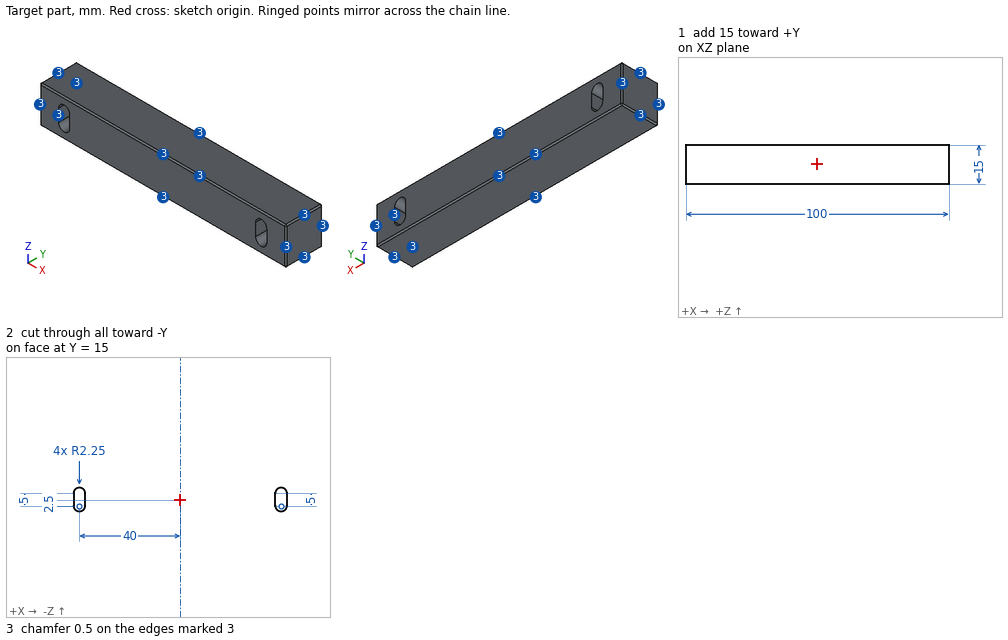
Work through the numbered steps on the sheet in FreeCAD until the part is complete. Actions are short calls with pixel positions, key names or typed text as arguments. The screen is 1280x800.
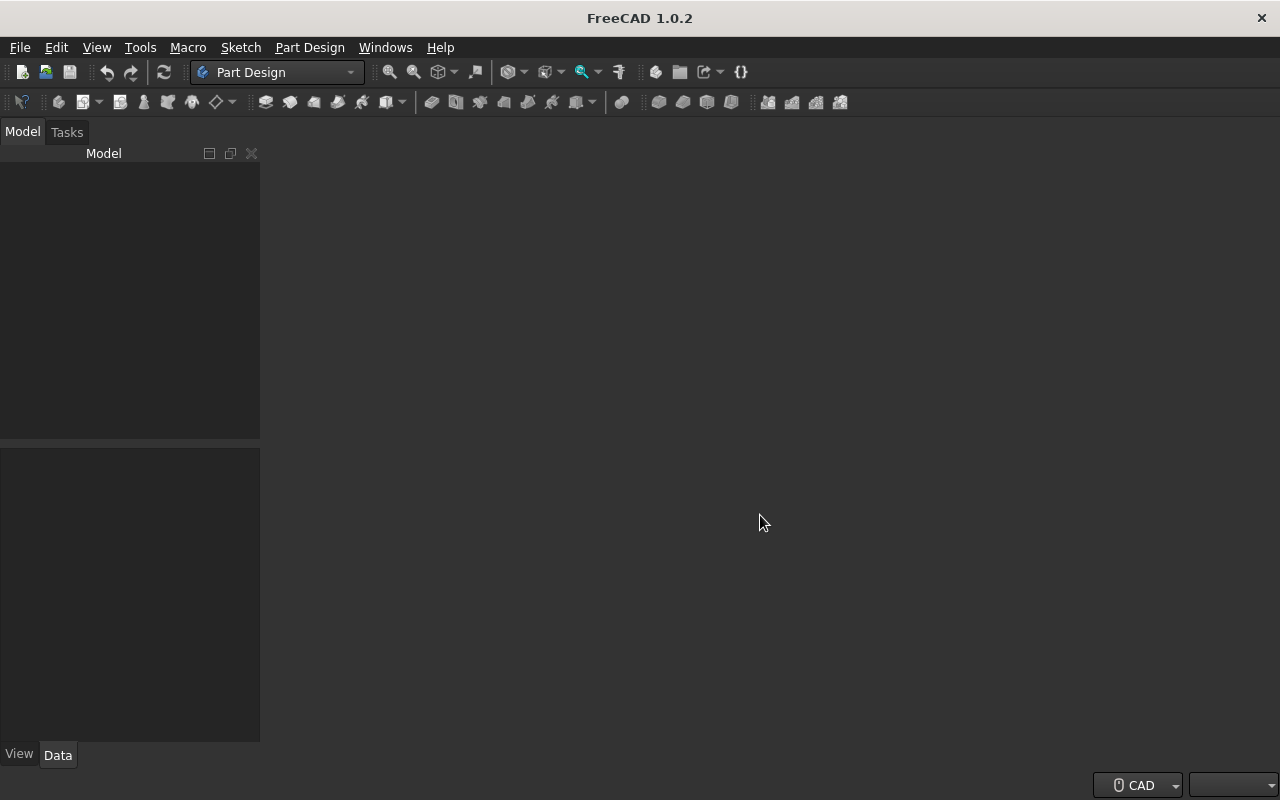
click(22, 72)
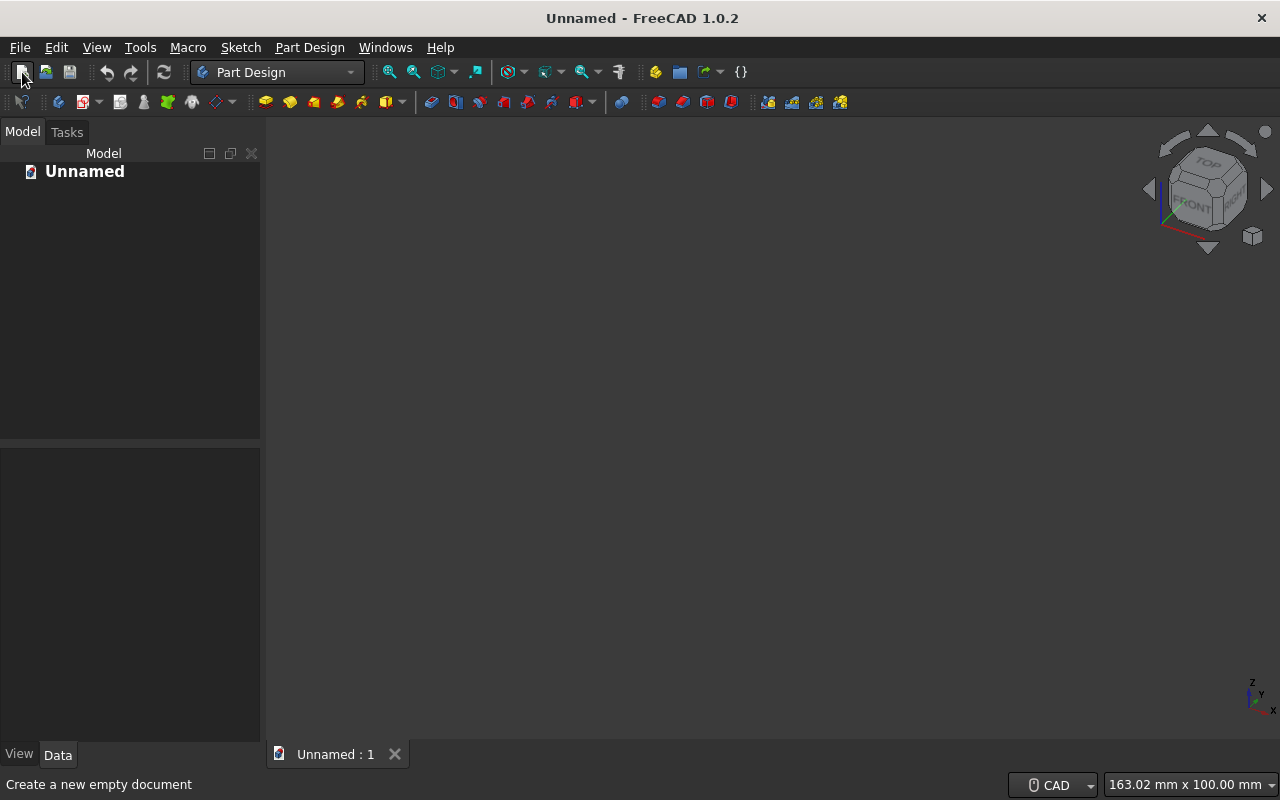
click(84, 102)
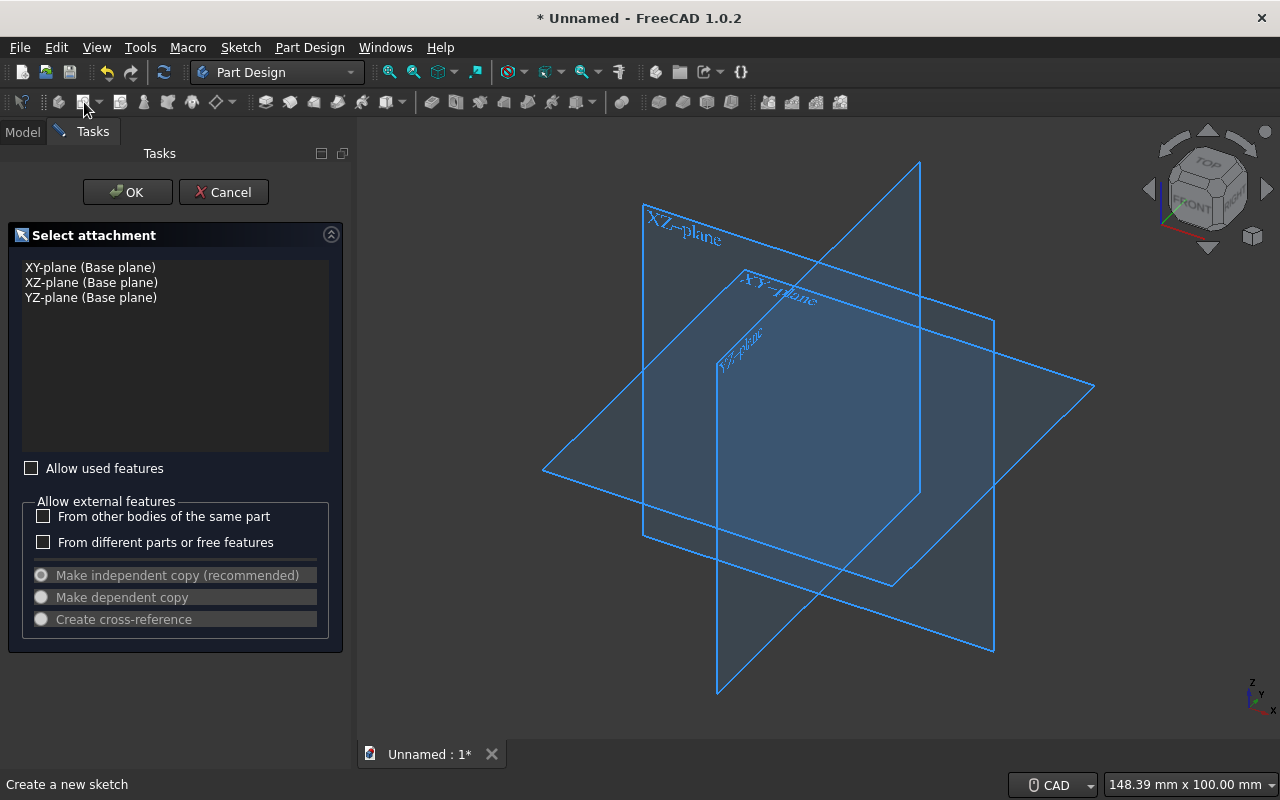
click(82, 282)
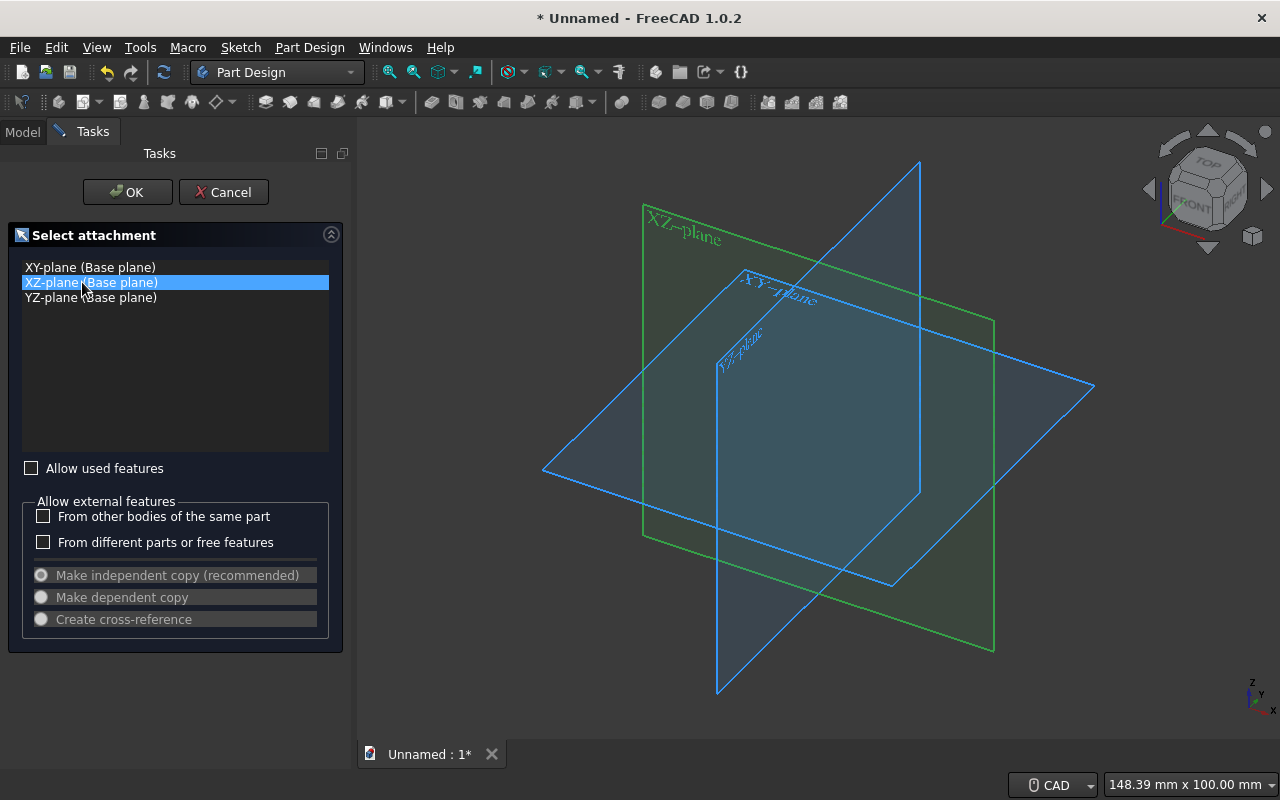
click(128, 192)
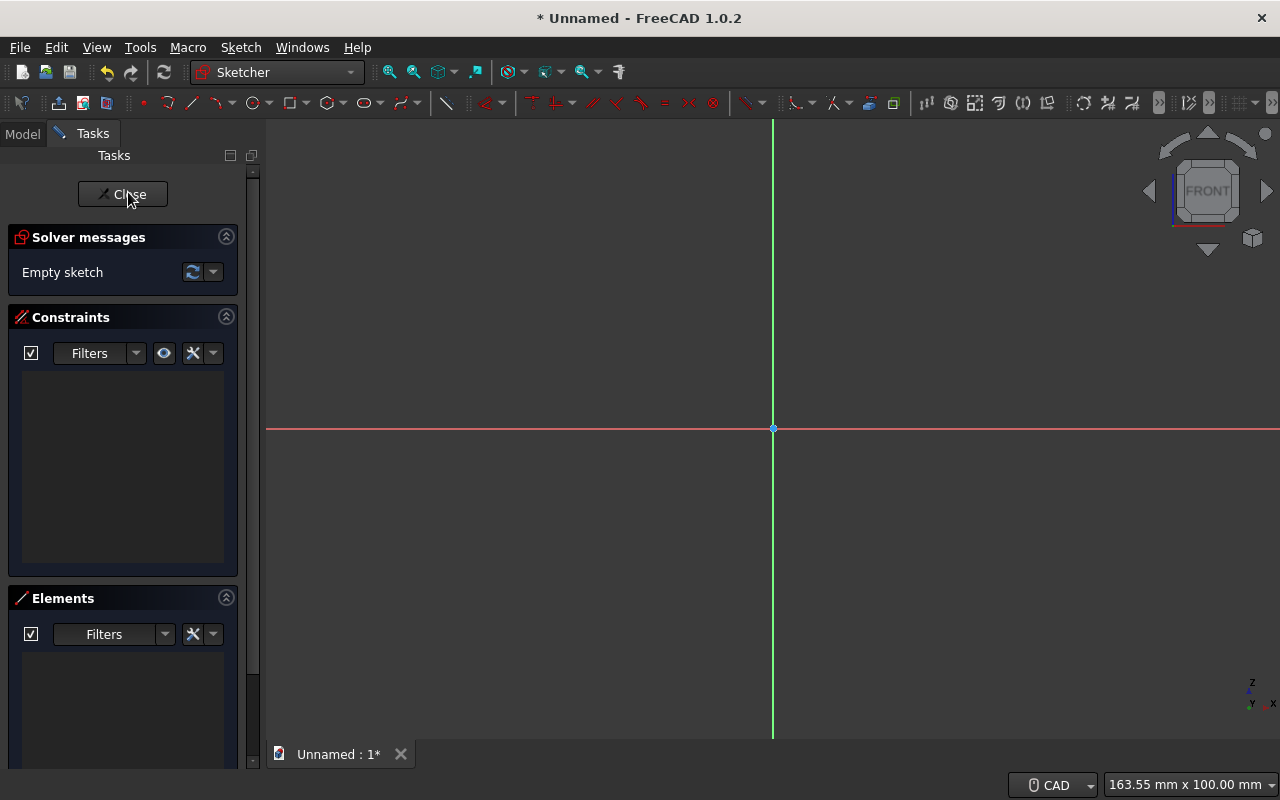
key(g)
key(v)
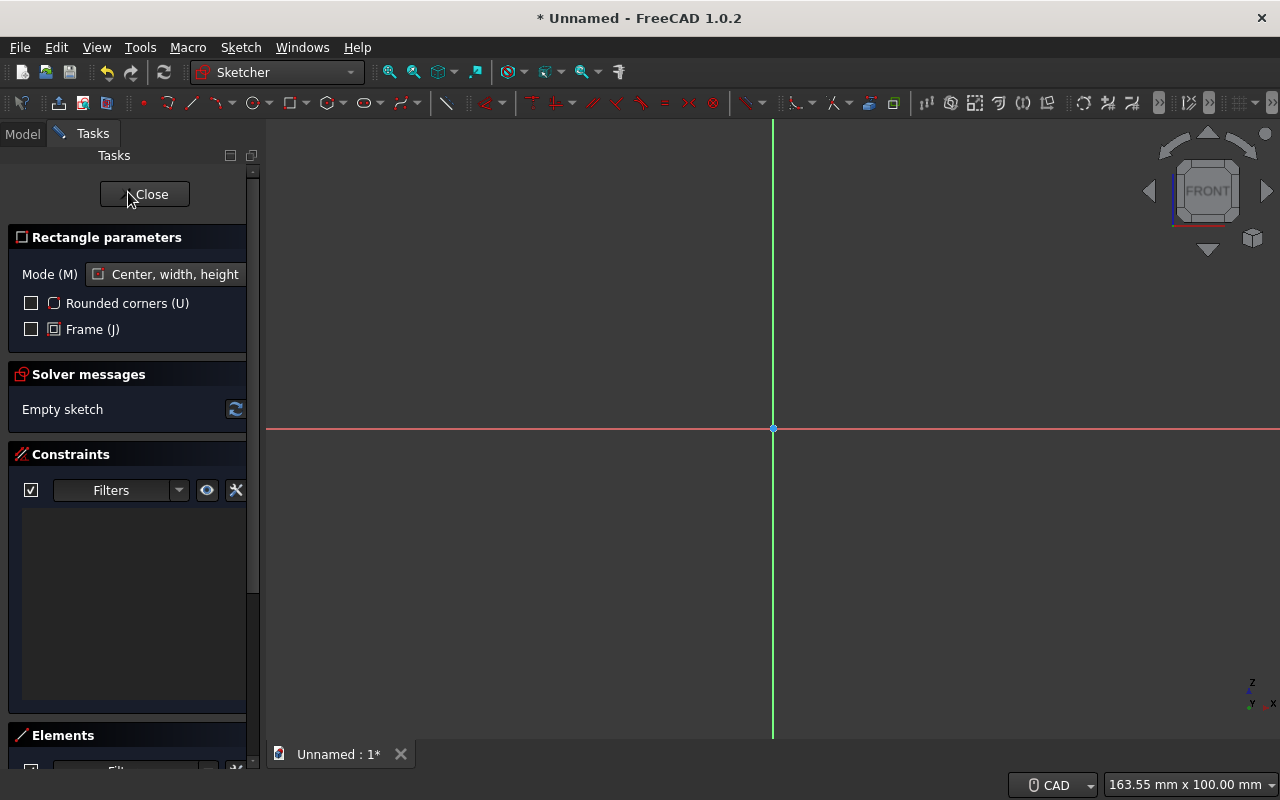
click(773, 429)
click(1083, 382)
key(Escape)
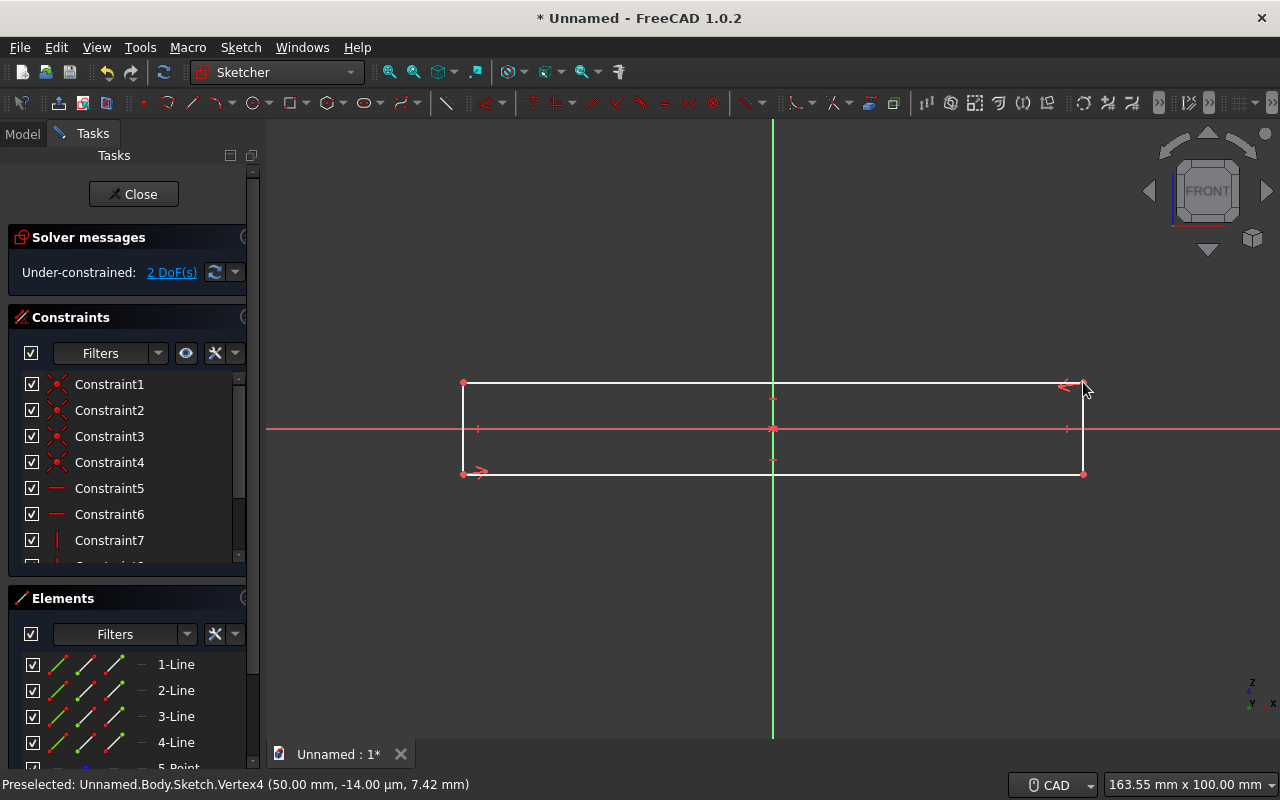
click(486, 104)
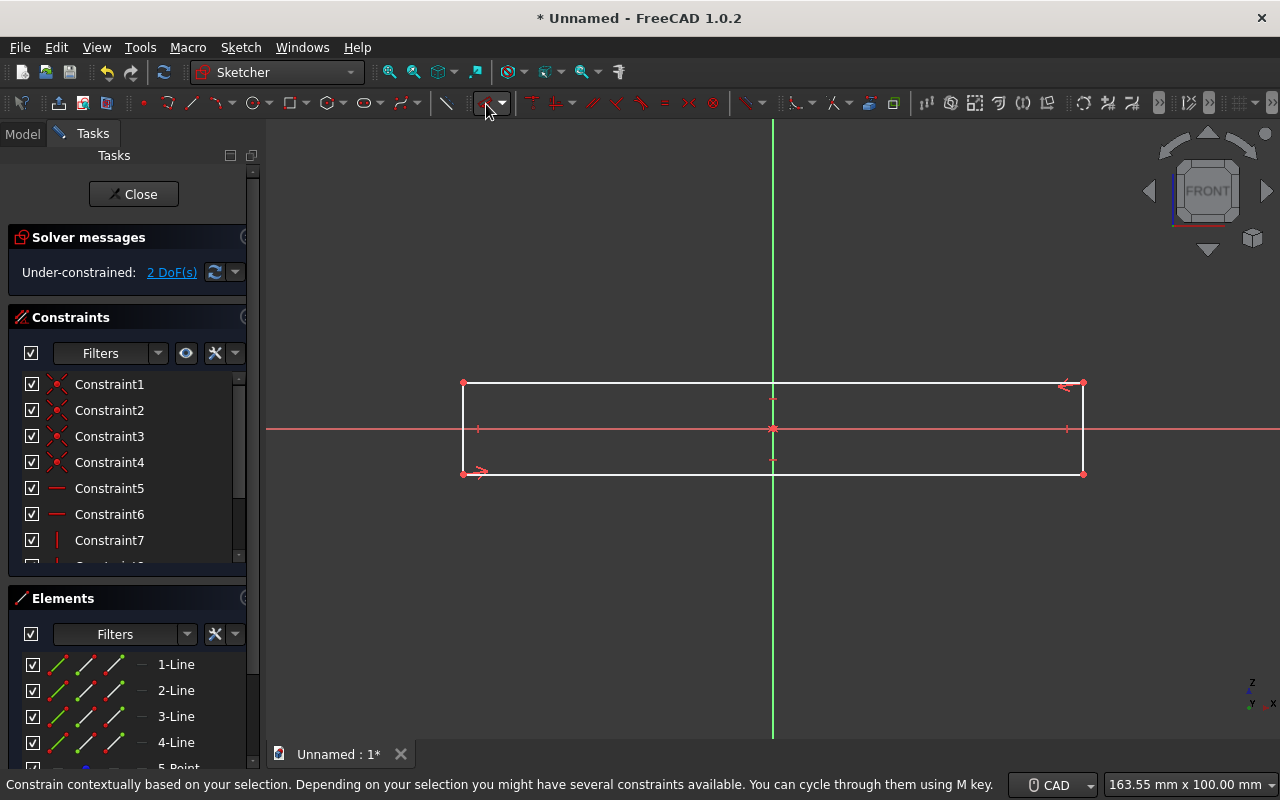
click(1083, 447)
click(1049, 408)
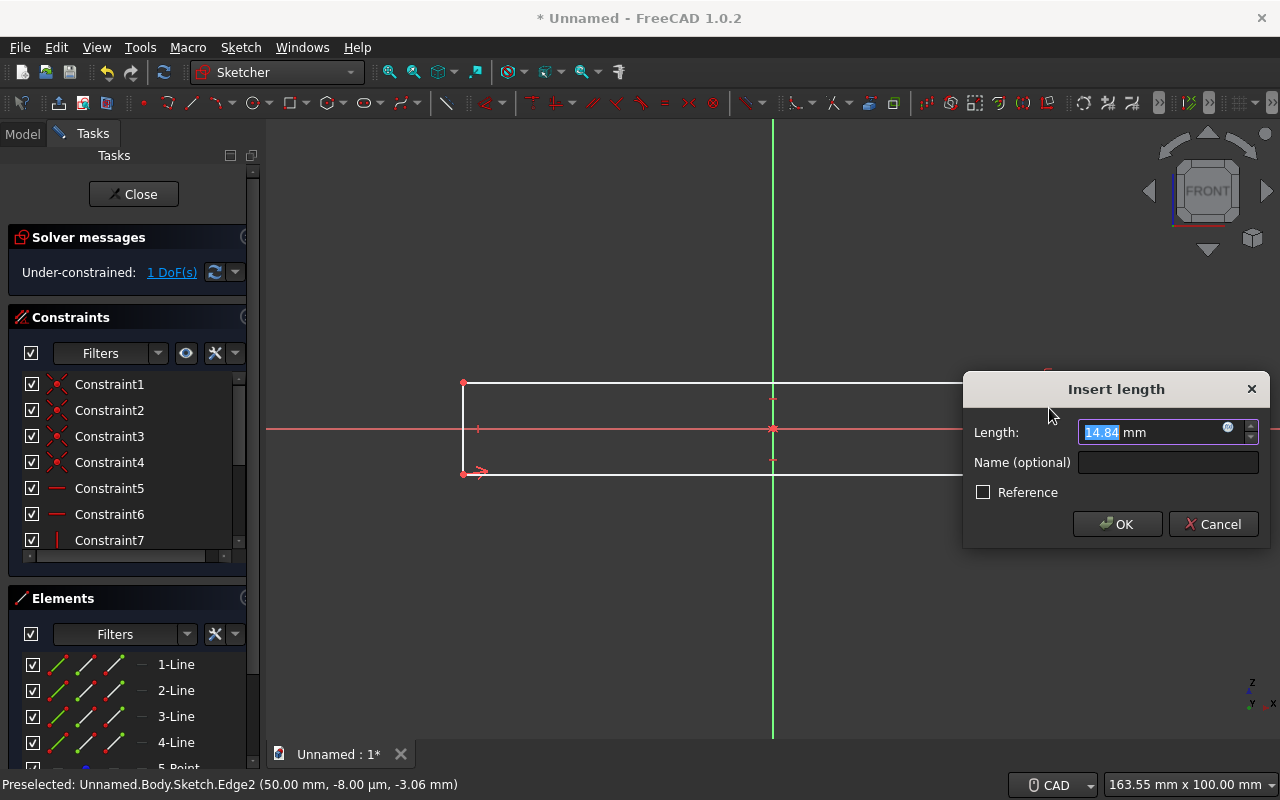
text(15)
key(Return)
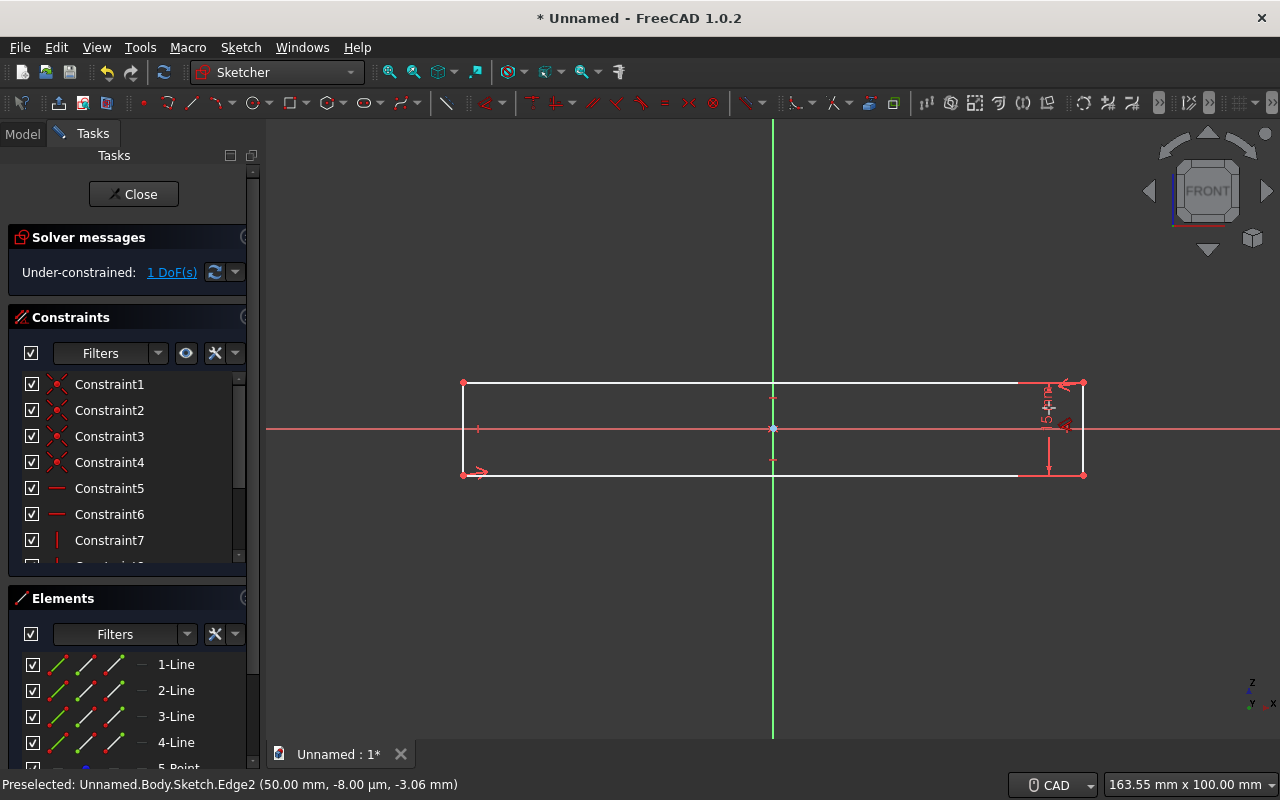
click(649, 476)
click(630, 510)